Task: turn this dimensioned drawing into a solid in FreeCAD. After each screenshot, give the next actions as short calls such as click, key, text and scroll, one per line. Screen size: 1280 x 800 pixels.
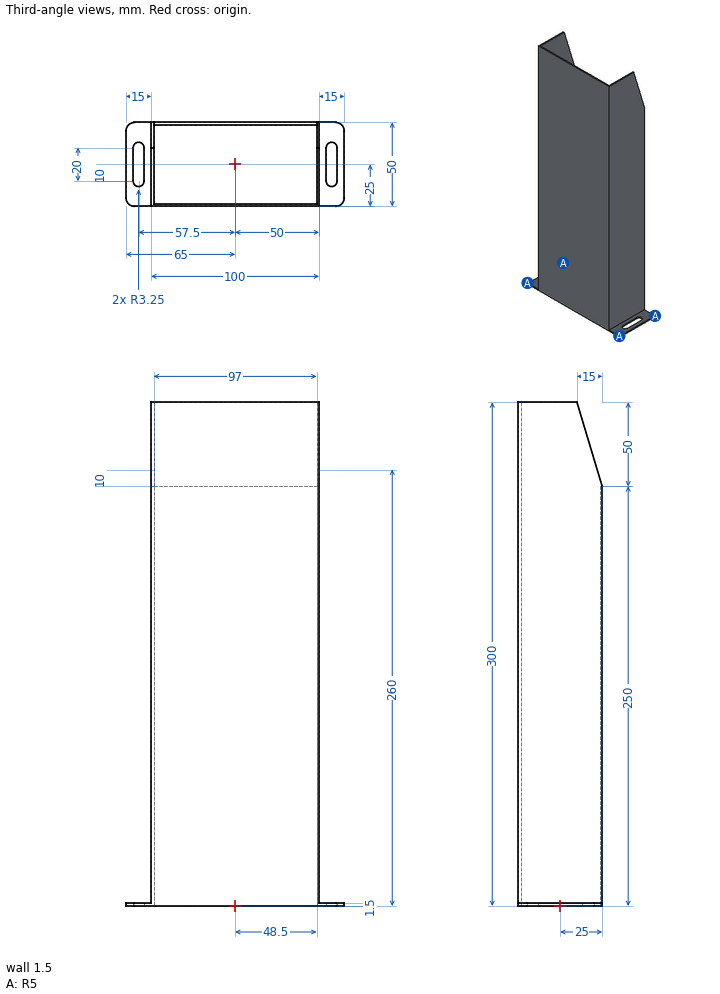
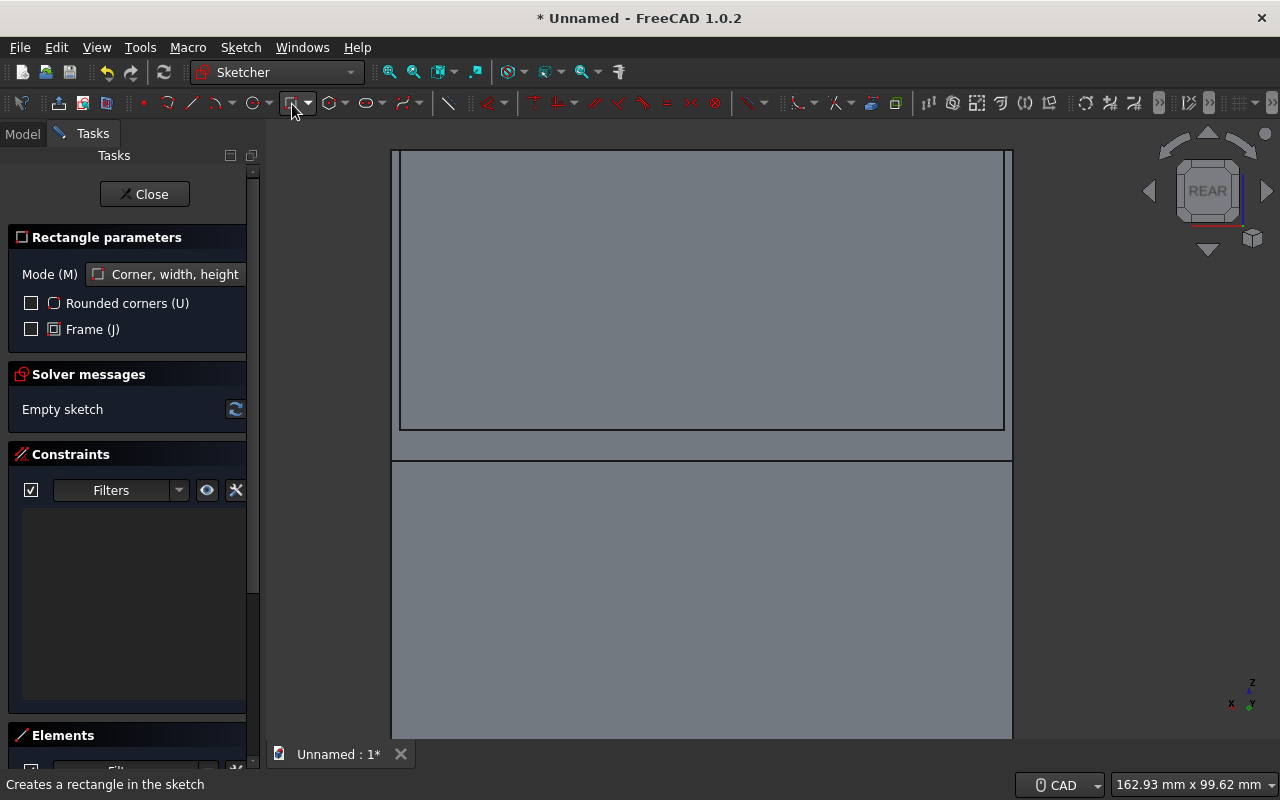
click(400, 399)
move(1004, 461)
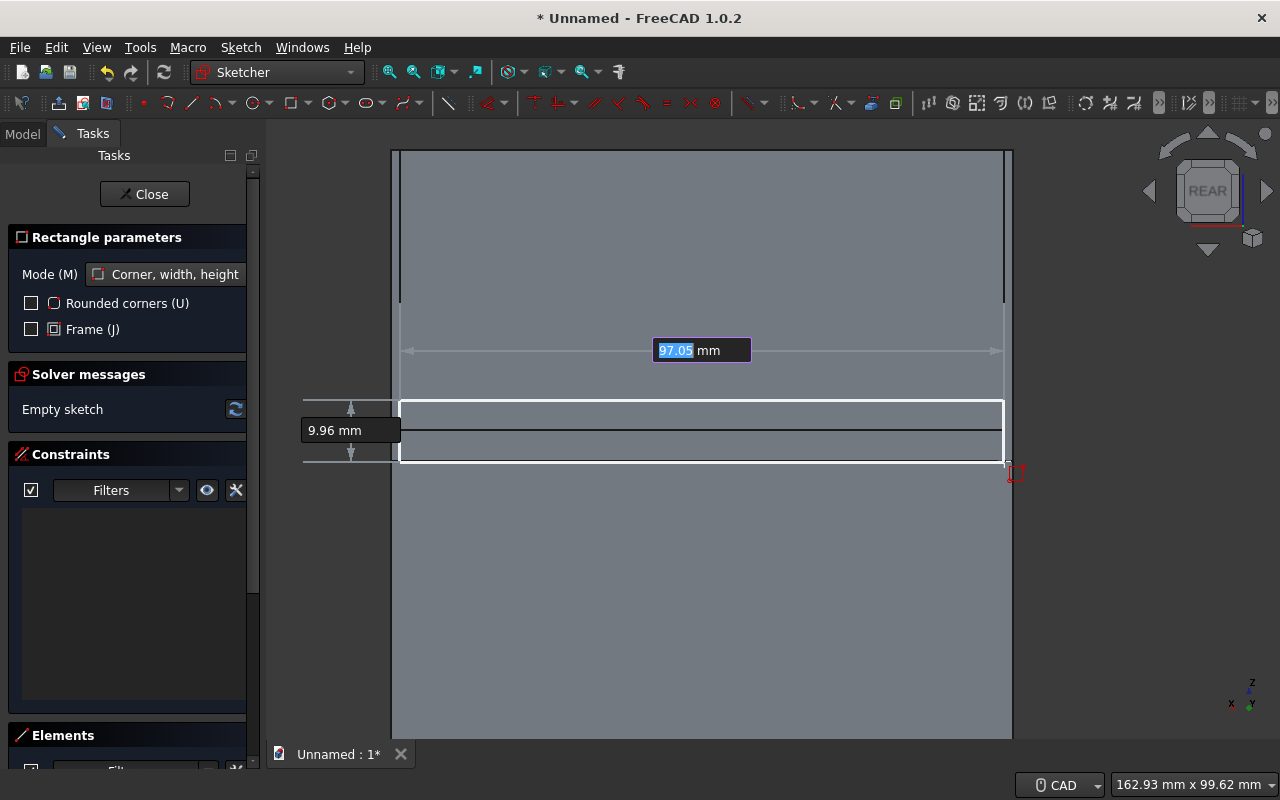
text(97)
key(Tab)
text(10)
key(Return)
key(Escape)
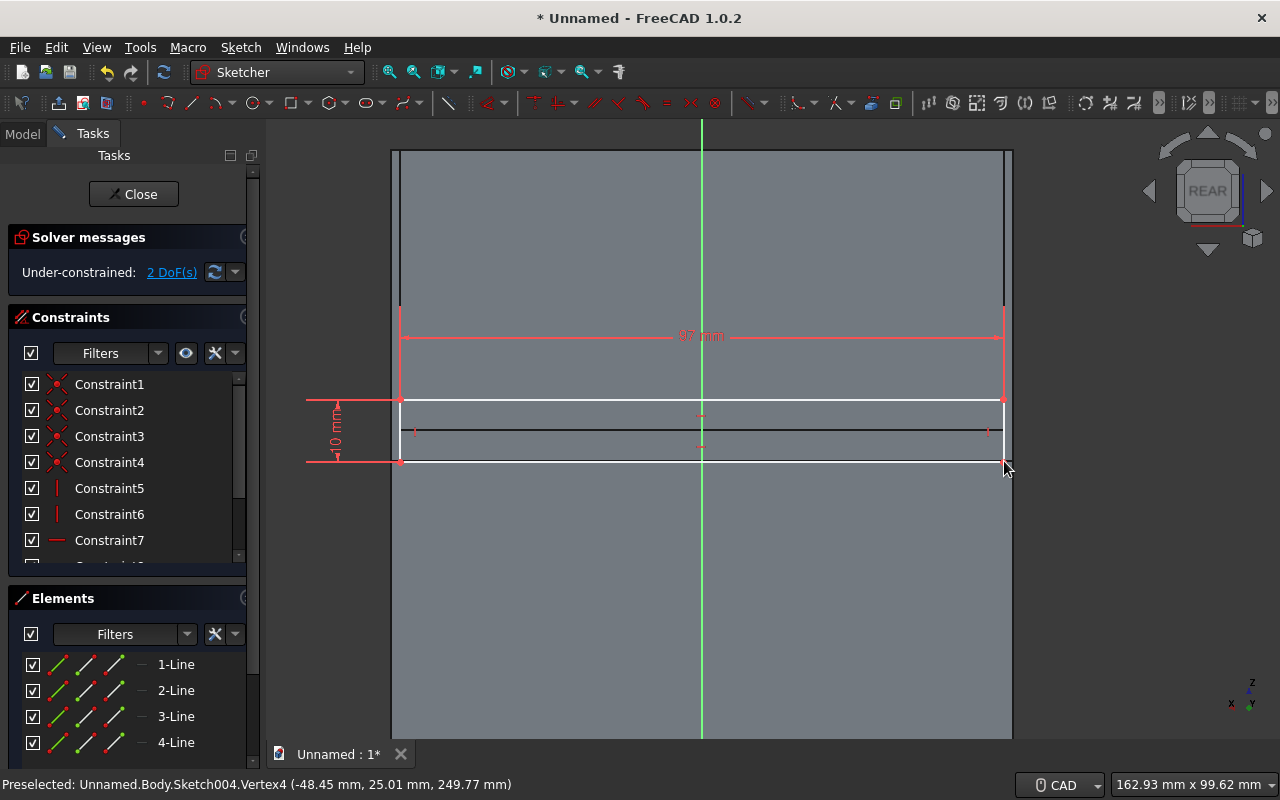
click(488, 104)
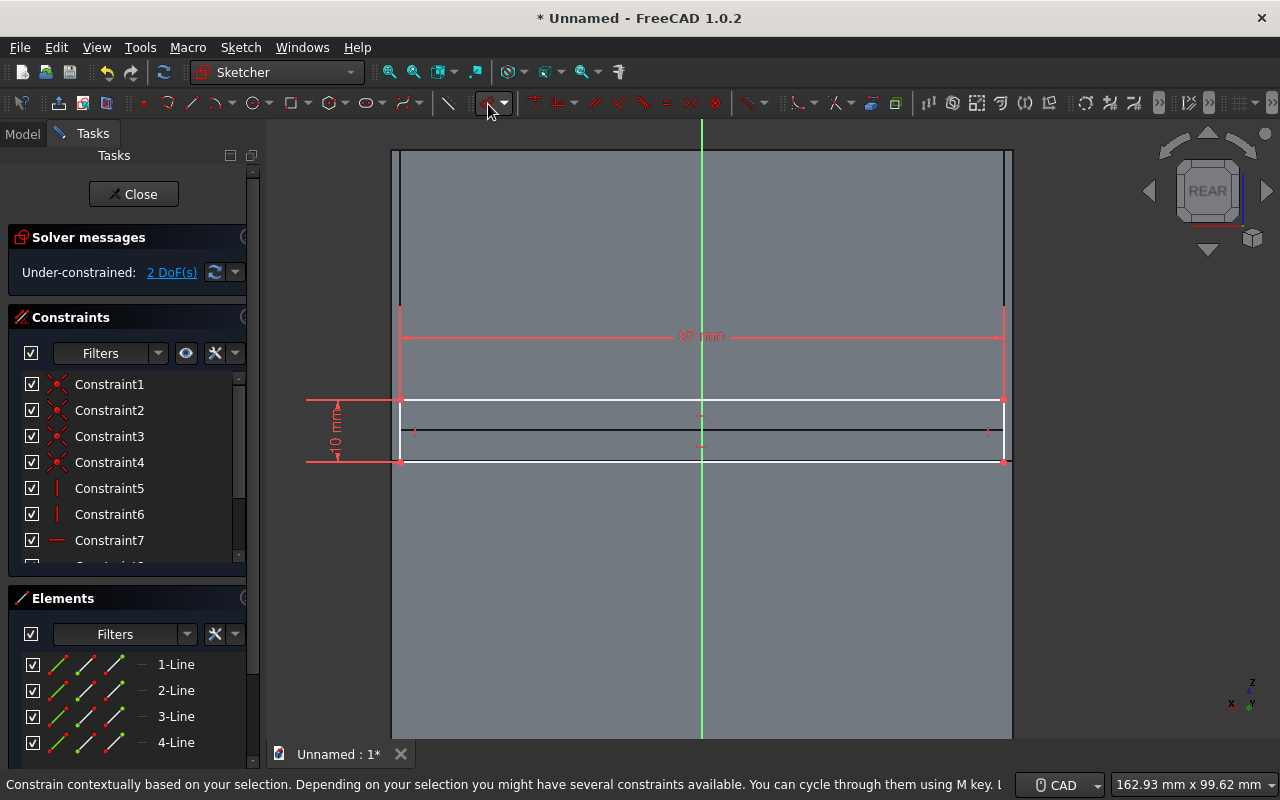
click(400, 400)
click(366, 556)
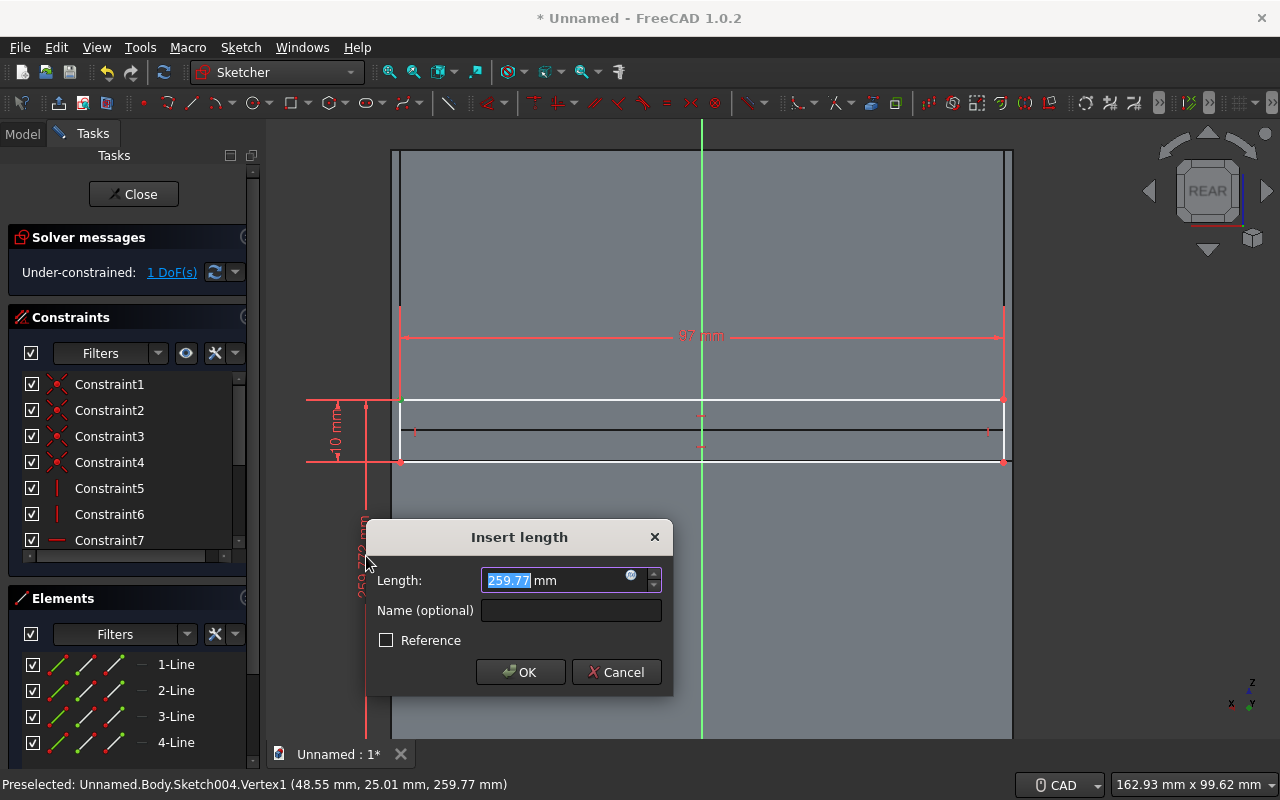
text(260)
key(Return)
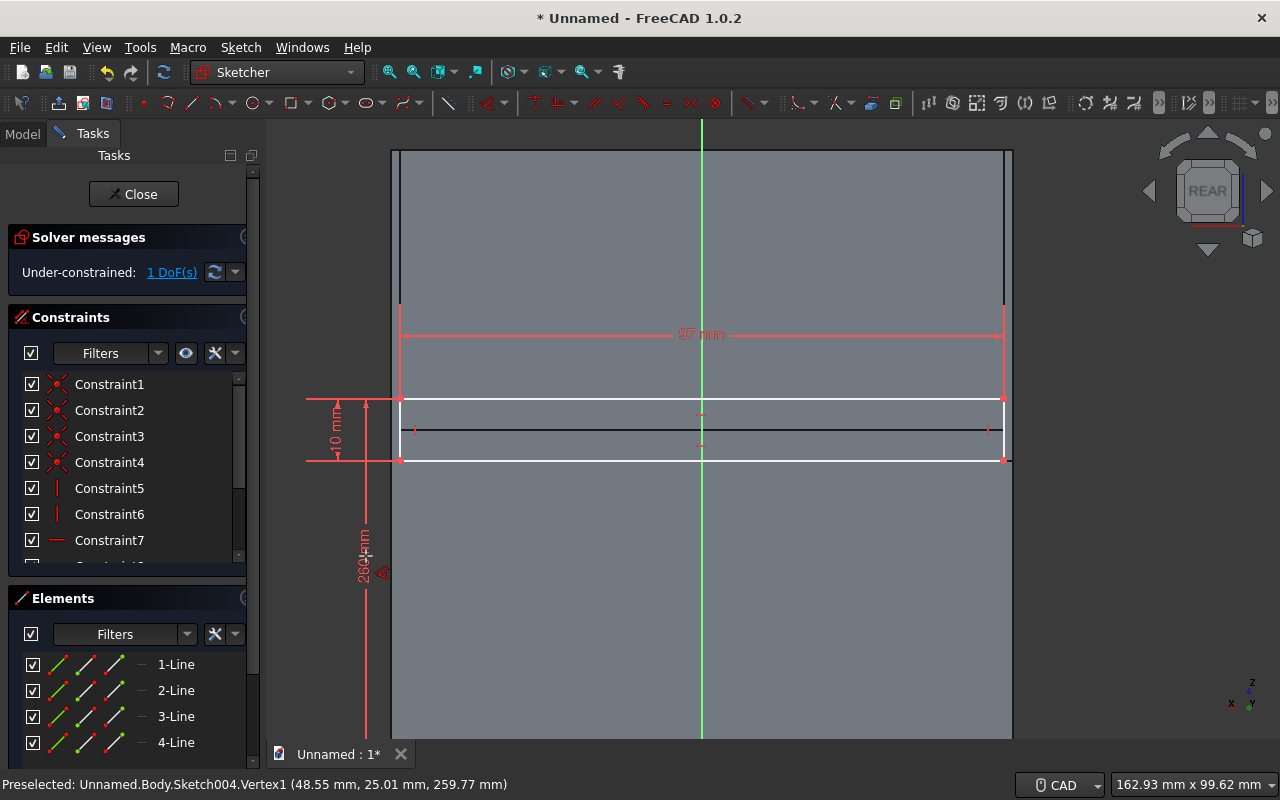
click(400, 399)
click(551, 365)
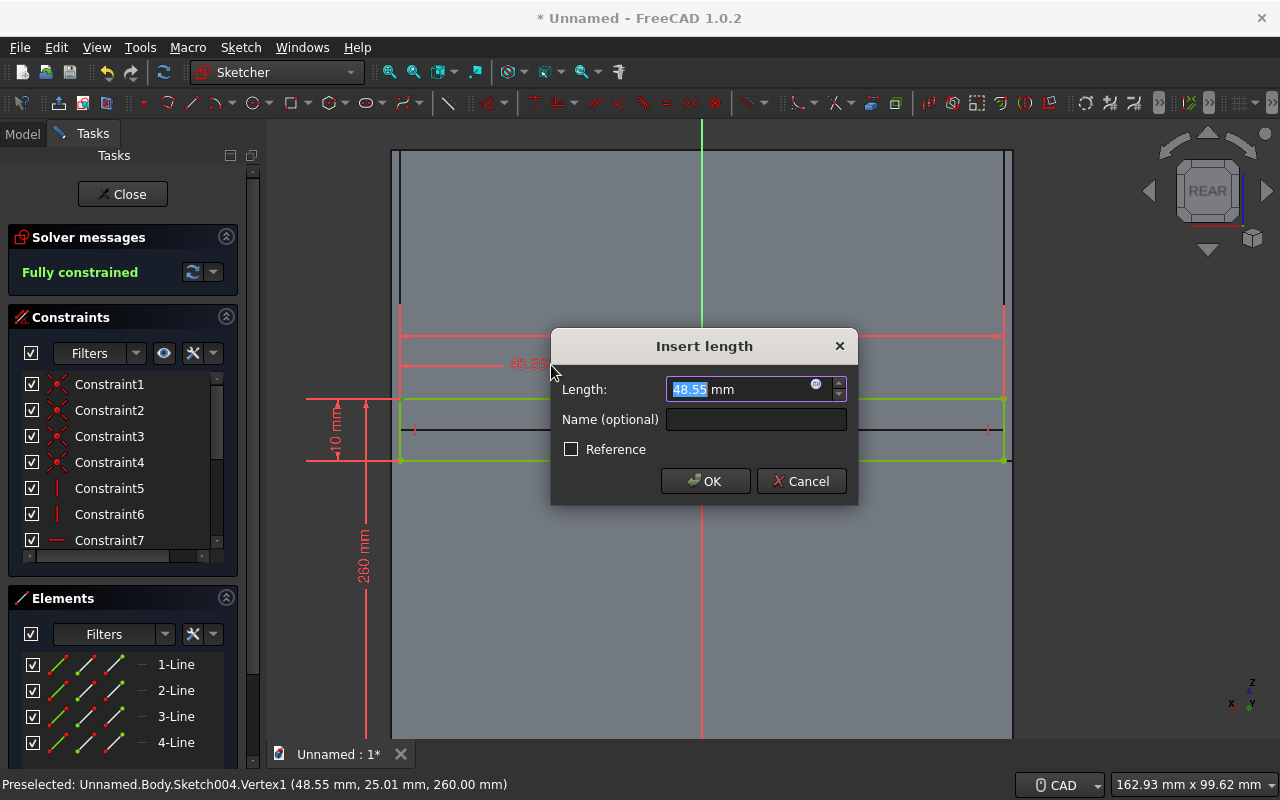
text(48.5)
key(Return)
key(Escape)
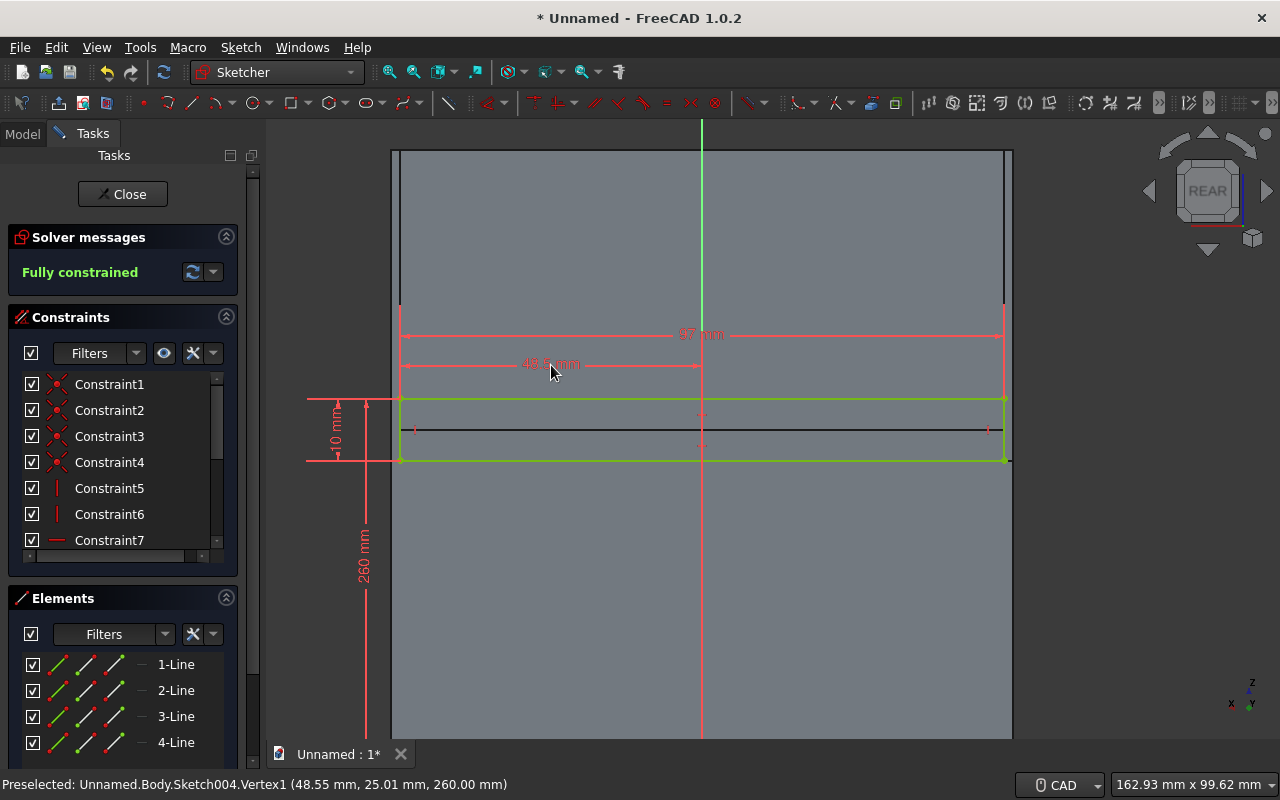
click(123, 194)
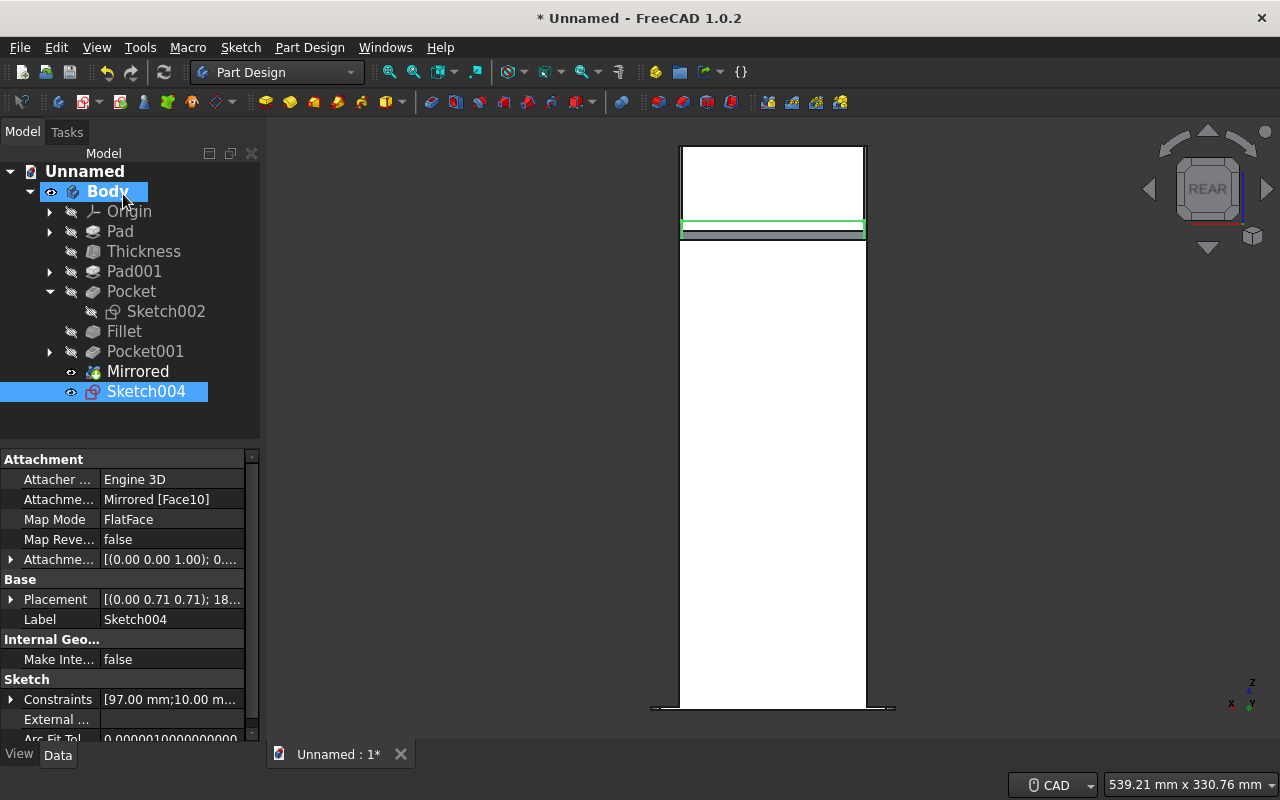
click(432, 102)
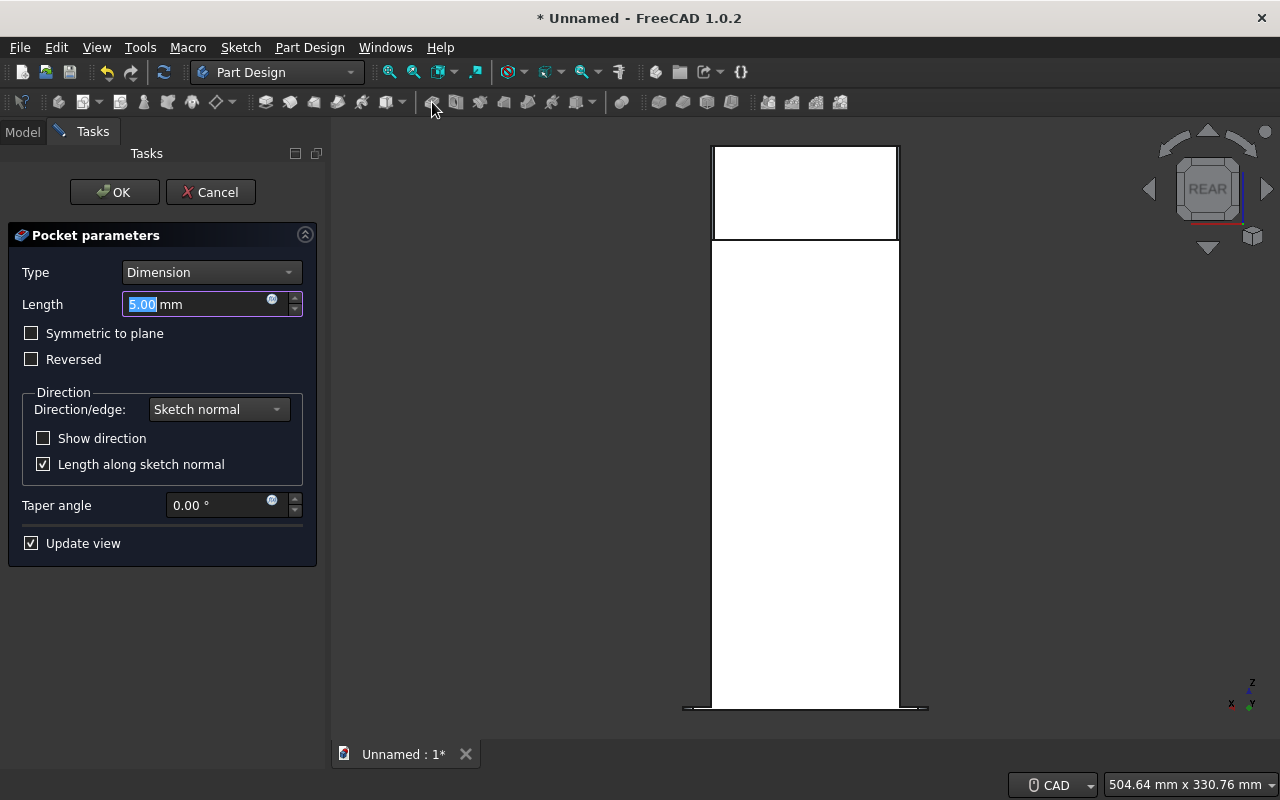
click(212, 272)